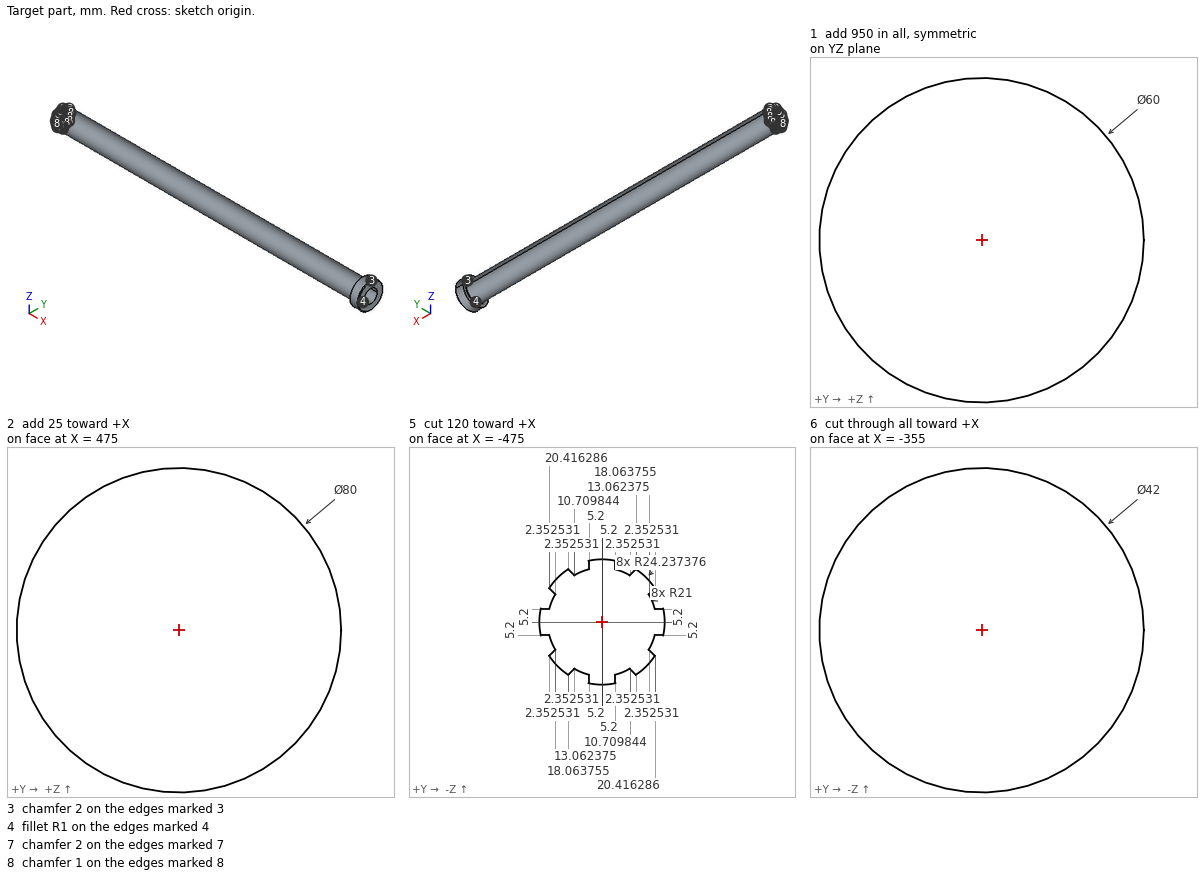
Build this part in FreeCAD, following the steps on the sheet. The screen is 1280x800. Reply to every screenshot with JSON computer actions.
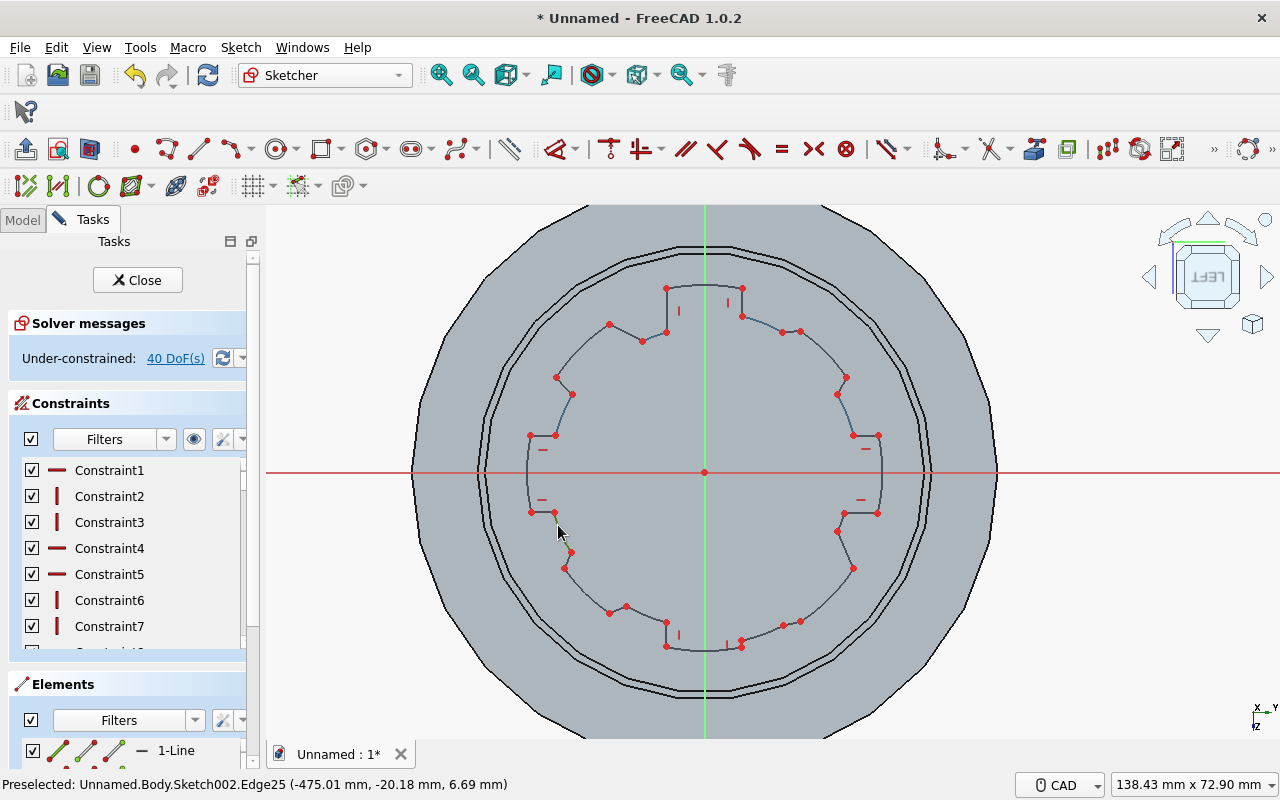
{"action": "left_click", "coordinate": [638, 612]}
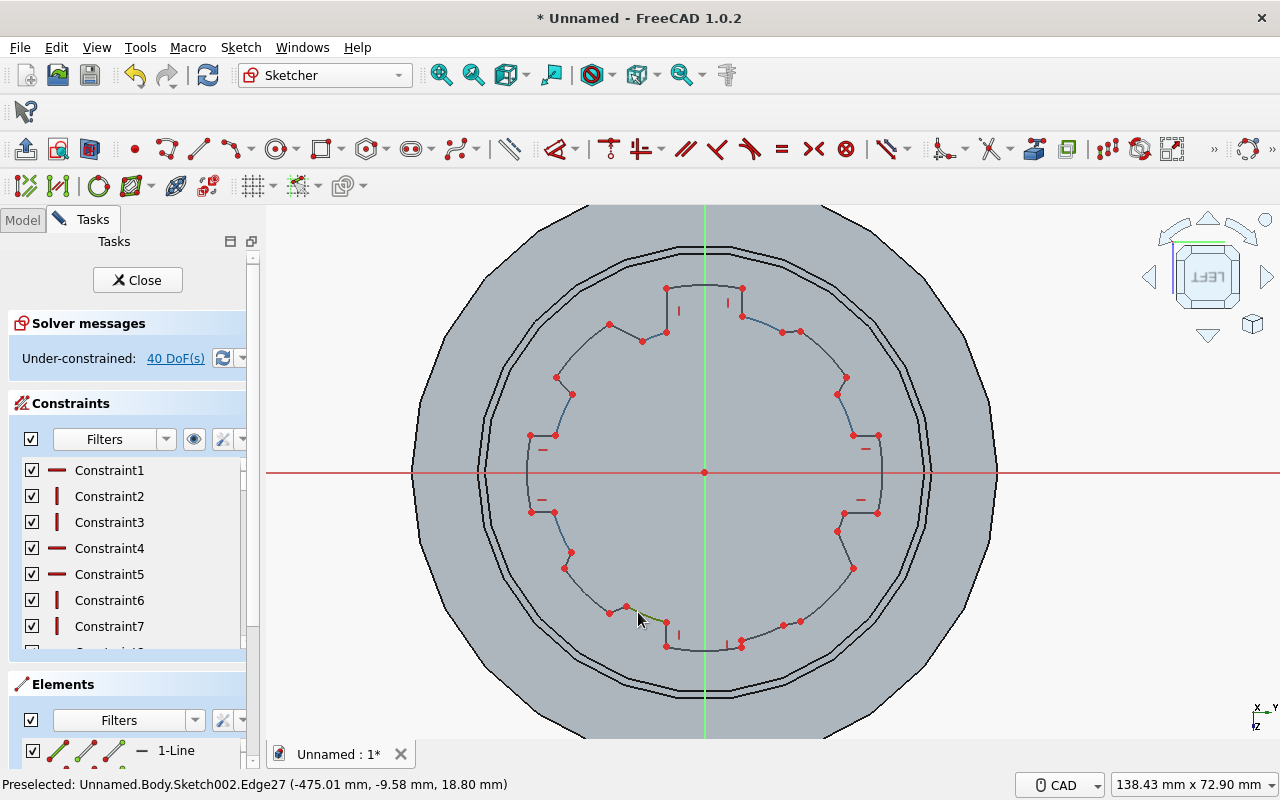
{"action": "left_click", "coordinate": [754, 637]}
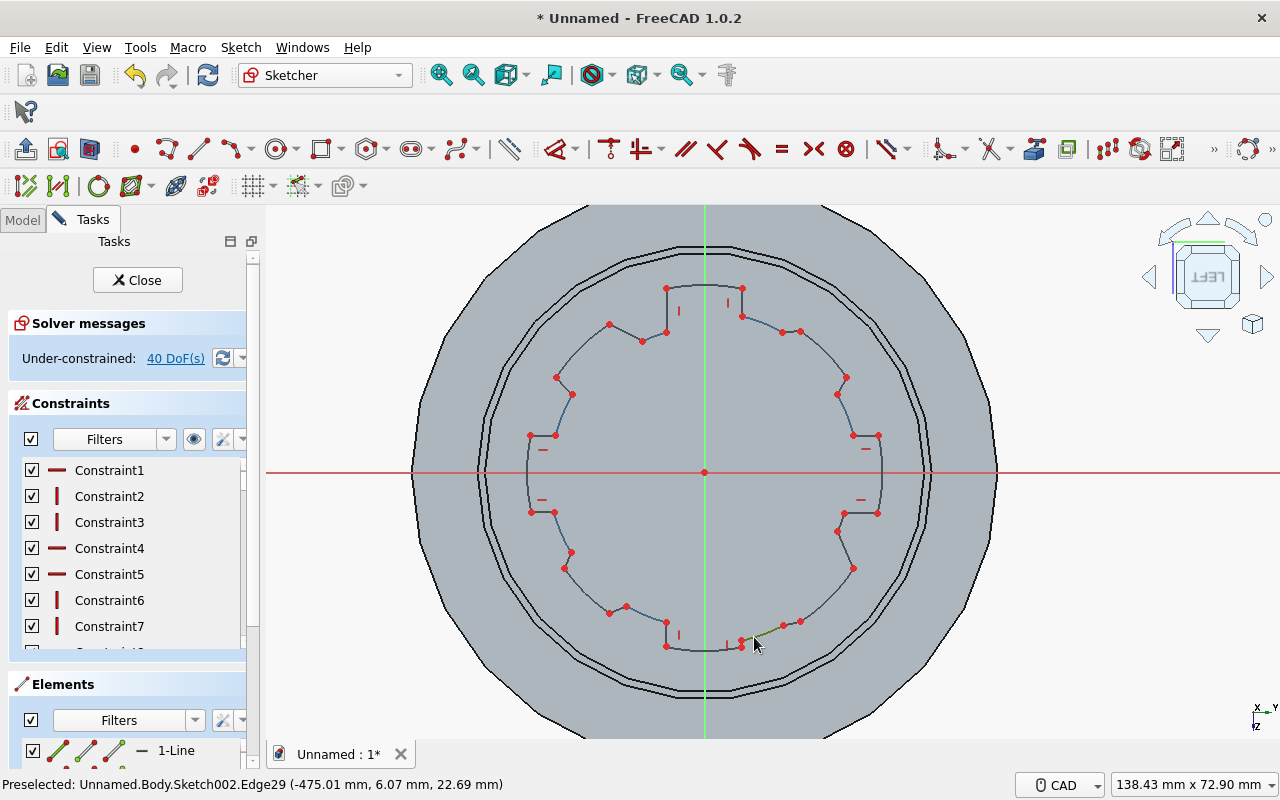
{"action": "scroll", "coordinate": [841, 523], "scroll_direction": "up", "scroll_amount": 2}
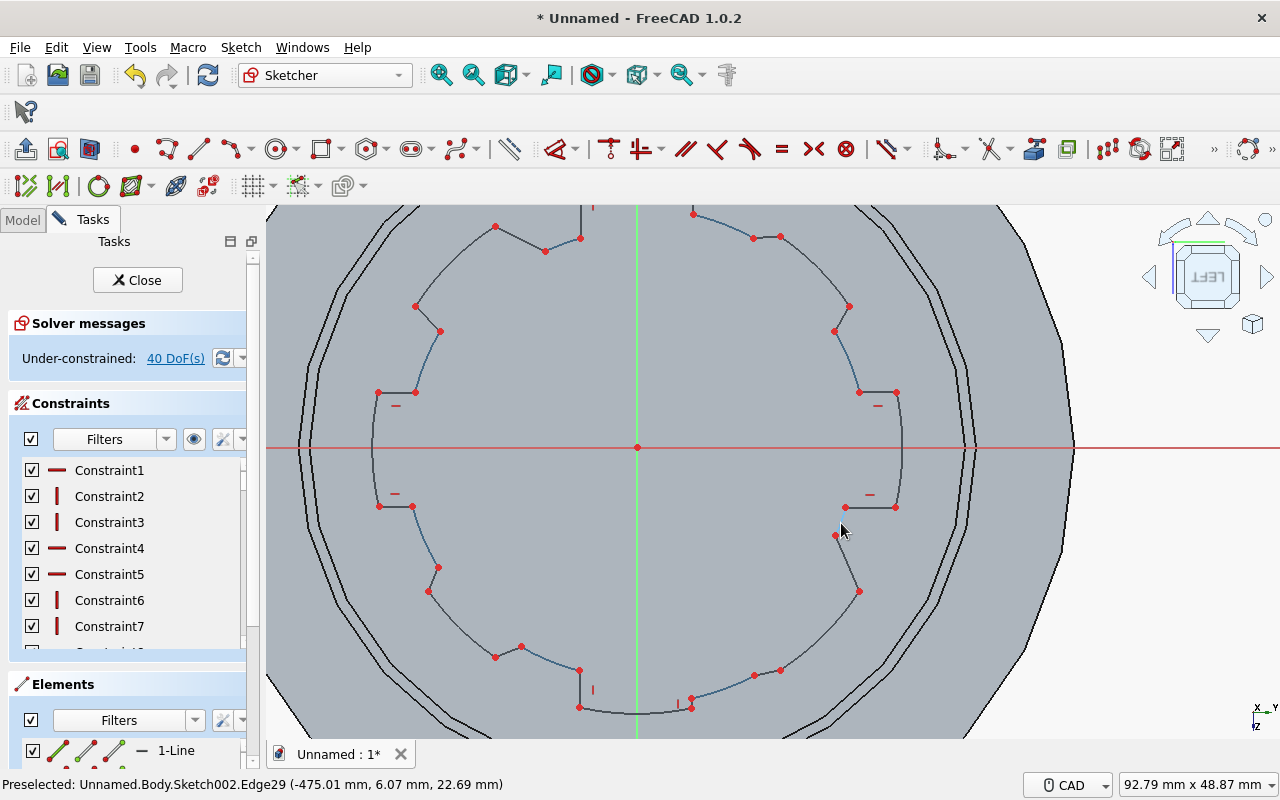
{"action": "left_click", "coordinate": [841, 522]}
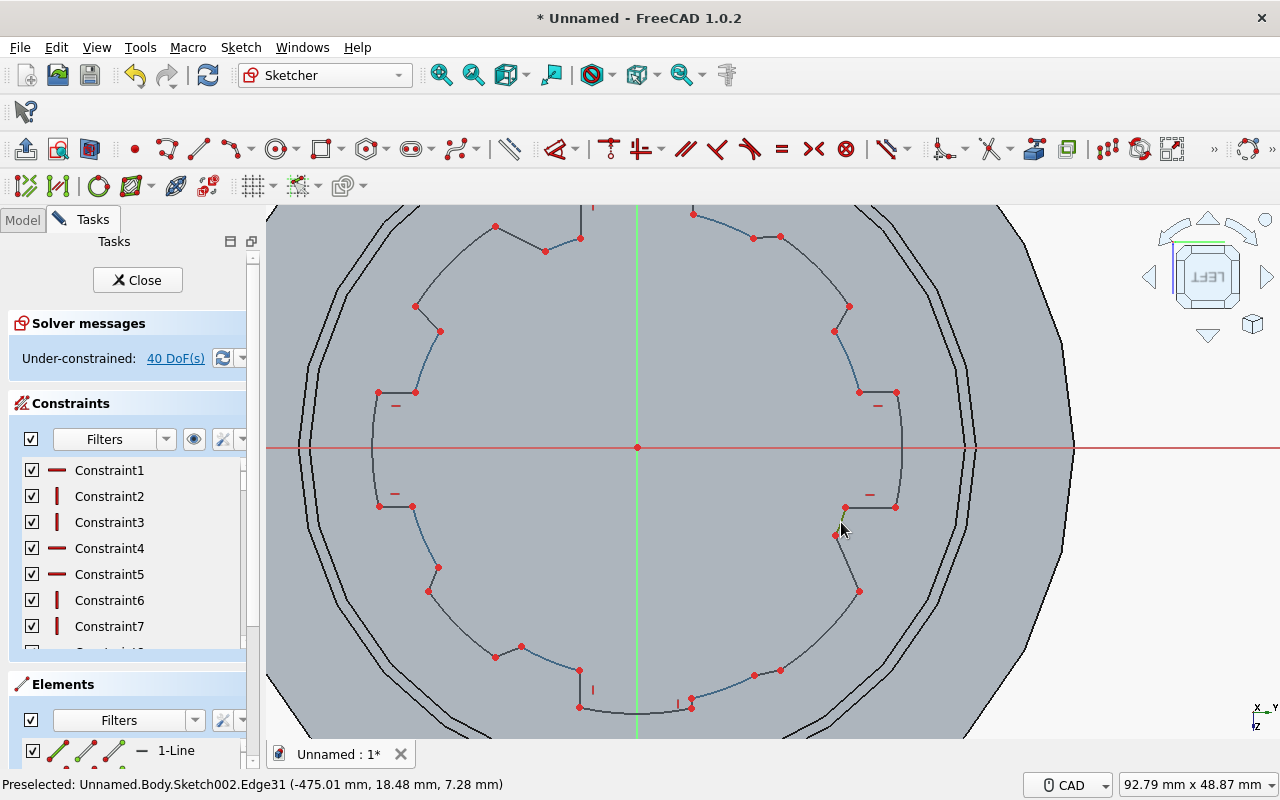
{"action": "key", "text": "e"}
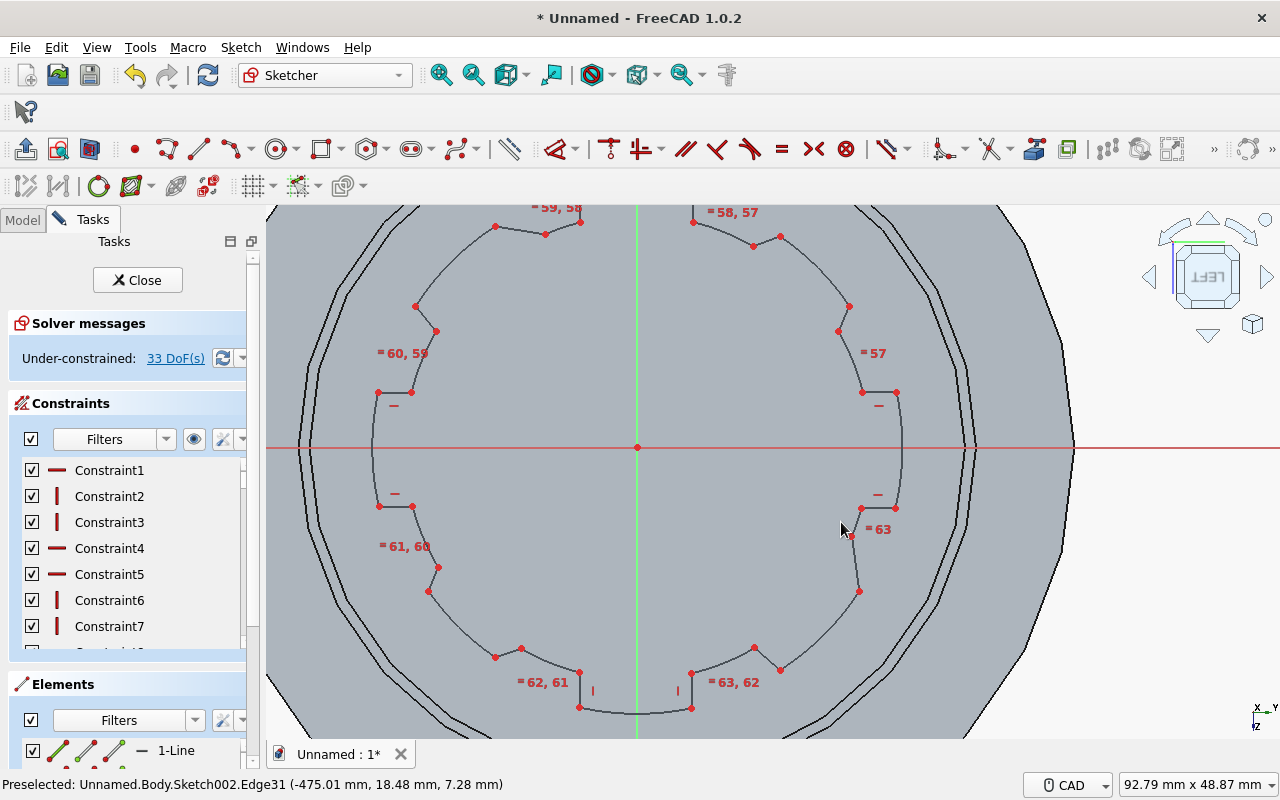
{"action": "left_click", "coordinate": [831, 282]}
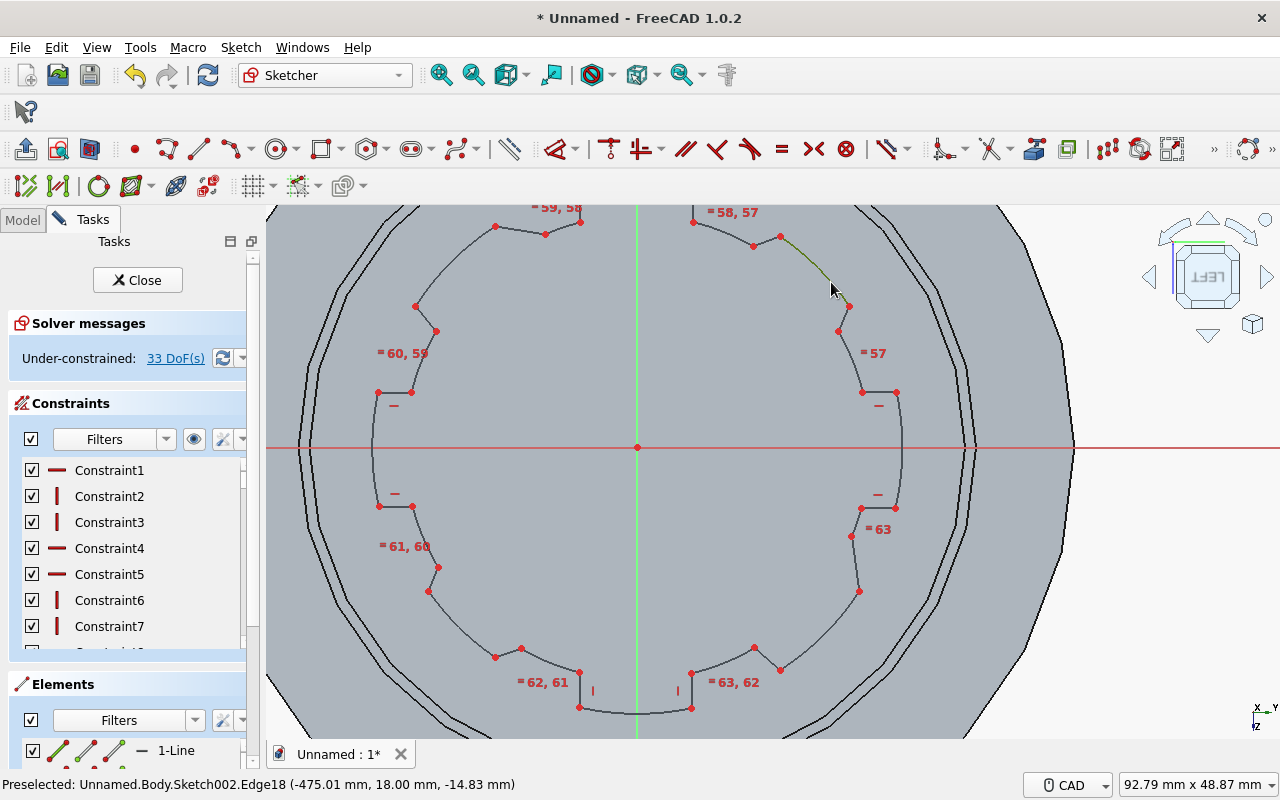
{"action": "scroll", "coordinate": [841, 522], "scroll_direction": "down", "scroll_amount": 2}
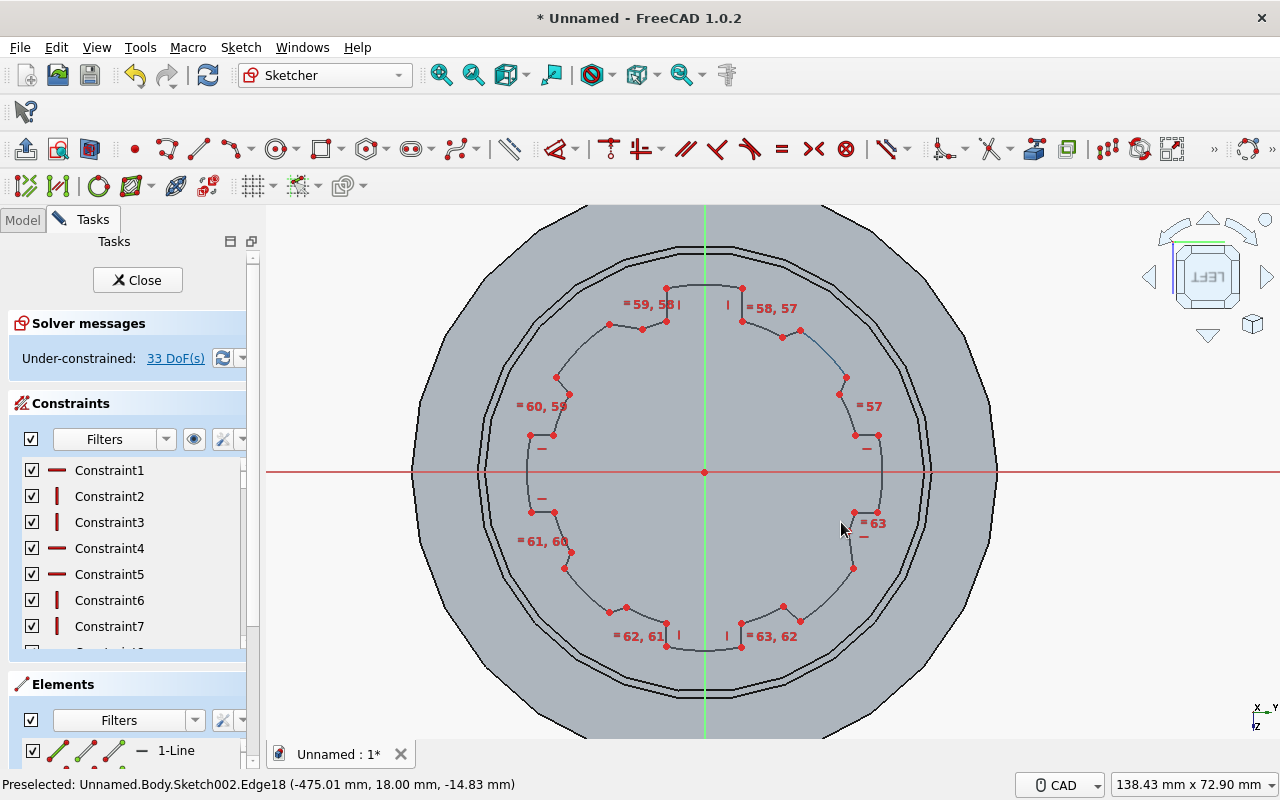
{"action": "left_click", "coordinate": [719, 285]}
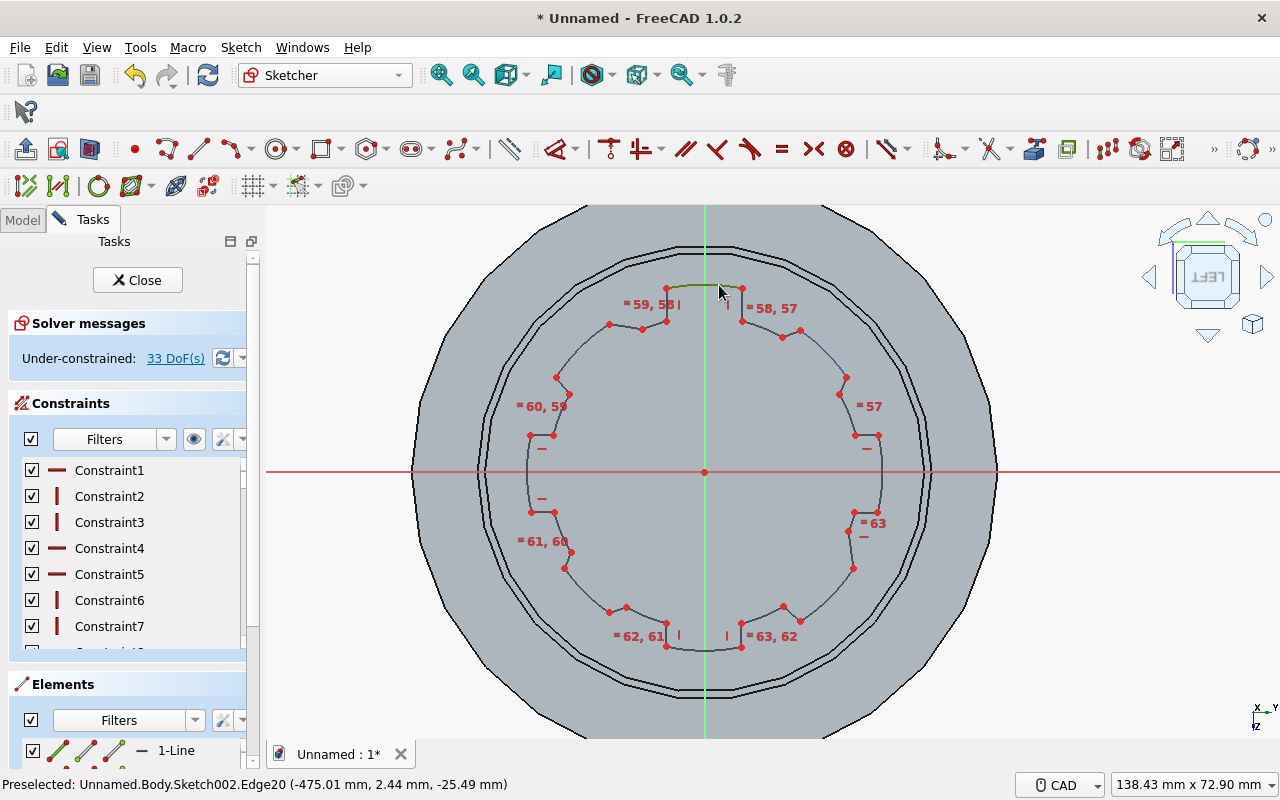
{"action": "left_click", "coordinate": [591, 338]}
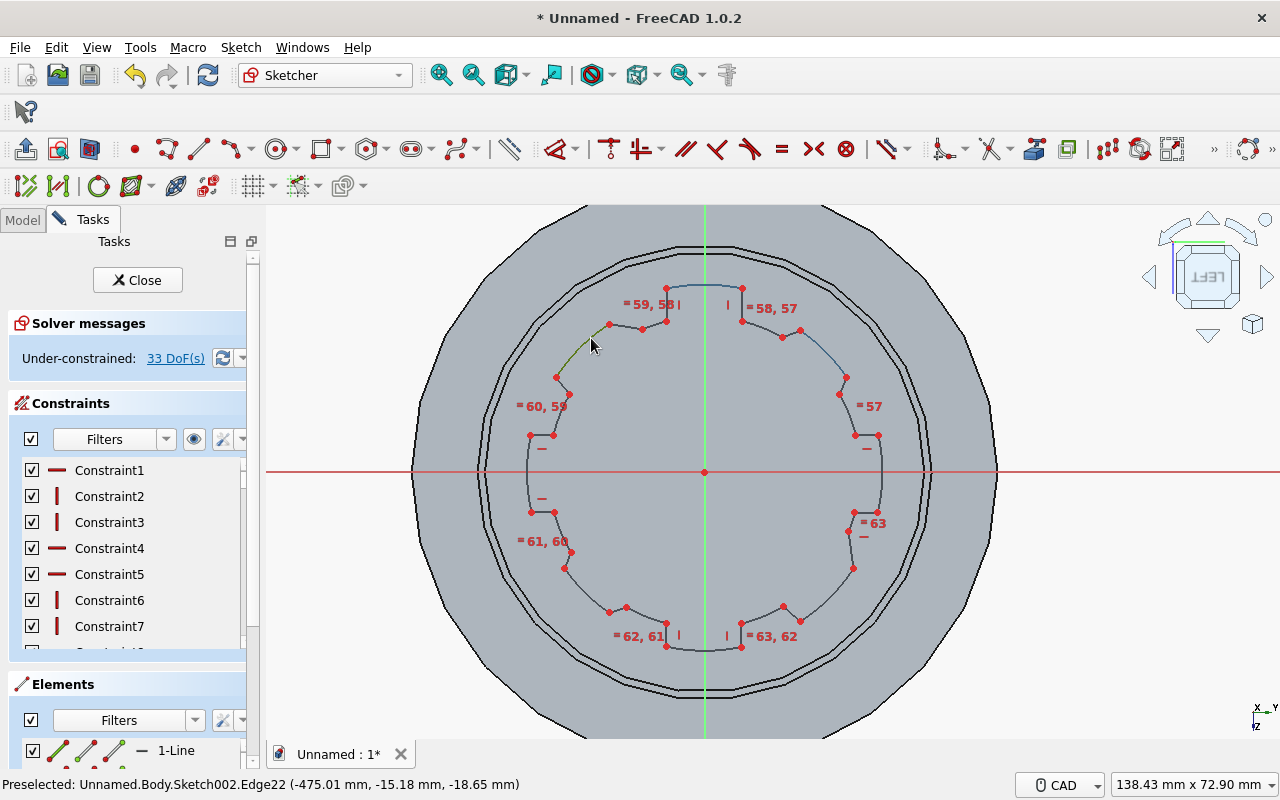
{"action": "left_click", "coordinate": [528, 458]}